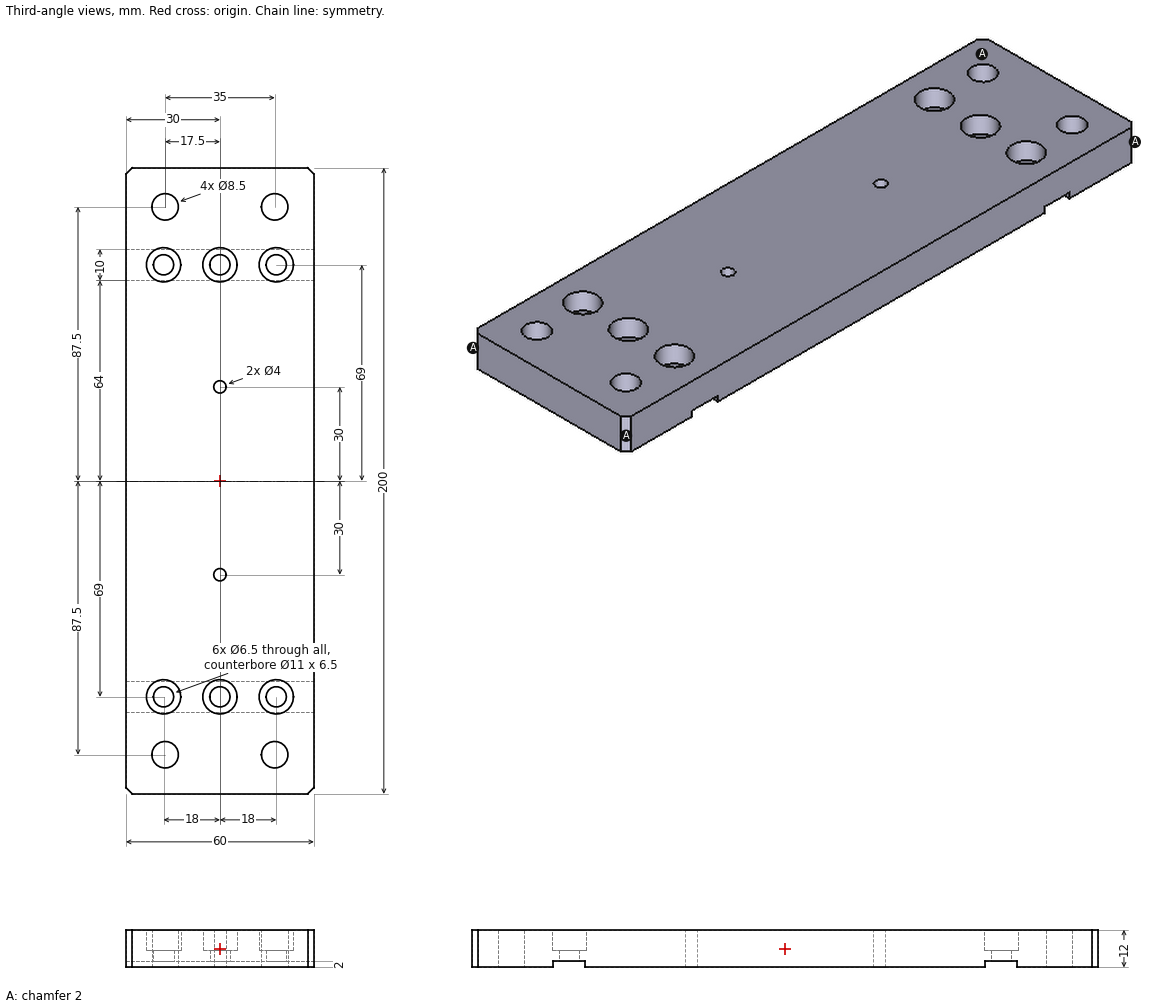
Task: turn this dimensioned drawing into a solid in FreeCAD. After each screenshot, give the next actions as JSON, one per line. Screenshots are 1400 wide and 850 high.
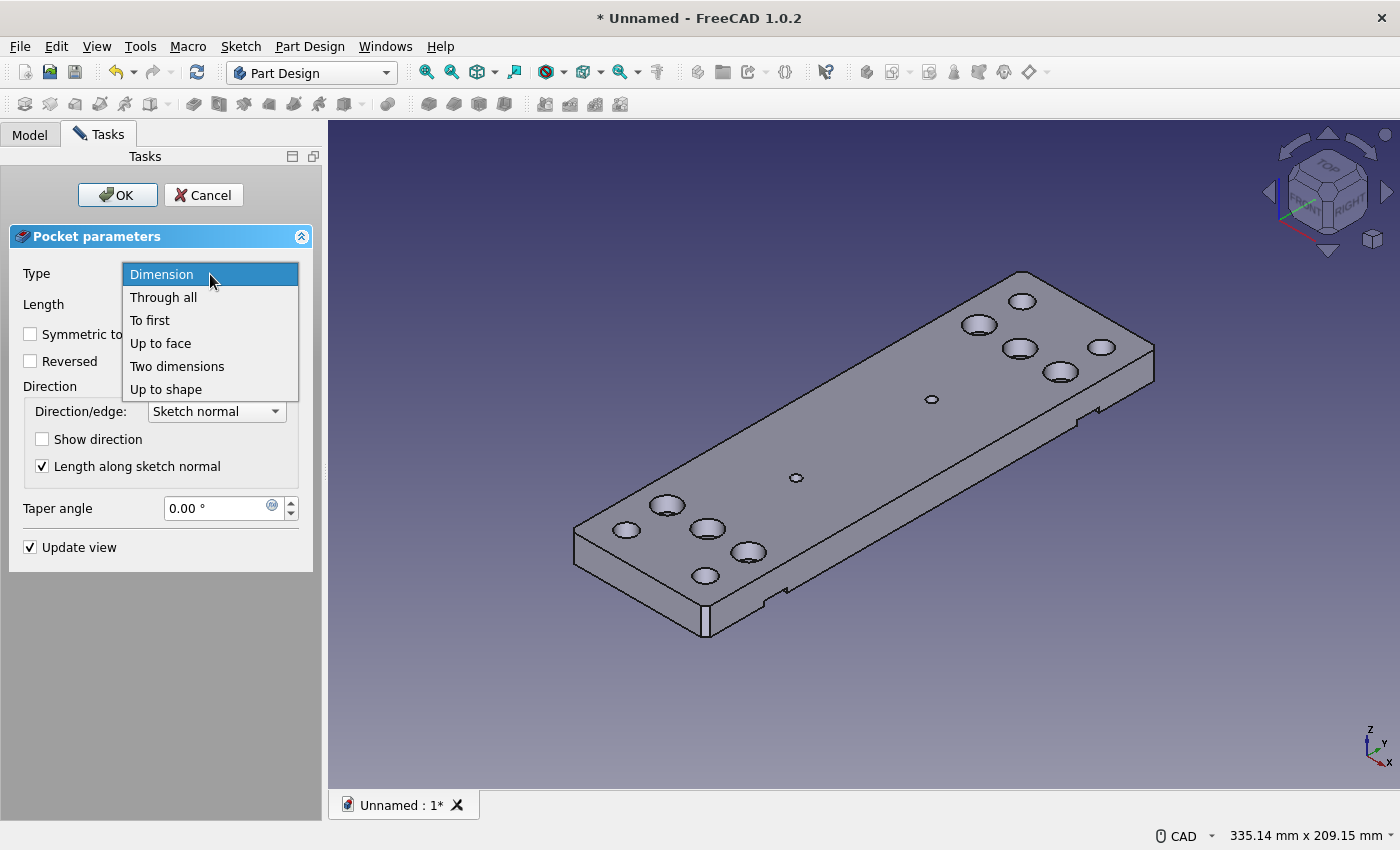
{"action": "left_click", "coordinate": [208, 298]}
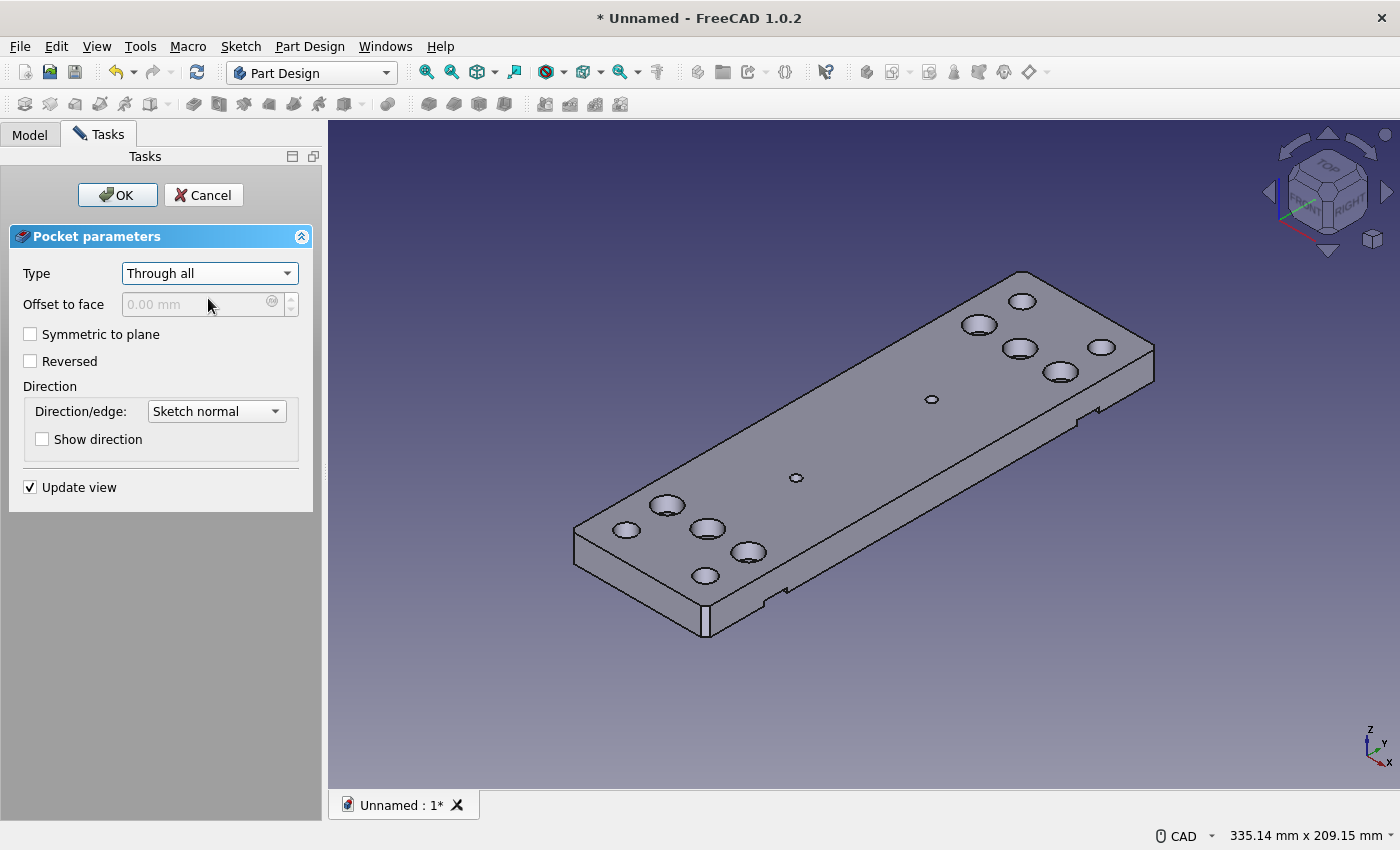
{"action": "left_click", "coordinate": [118, 195]}